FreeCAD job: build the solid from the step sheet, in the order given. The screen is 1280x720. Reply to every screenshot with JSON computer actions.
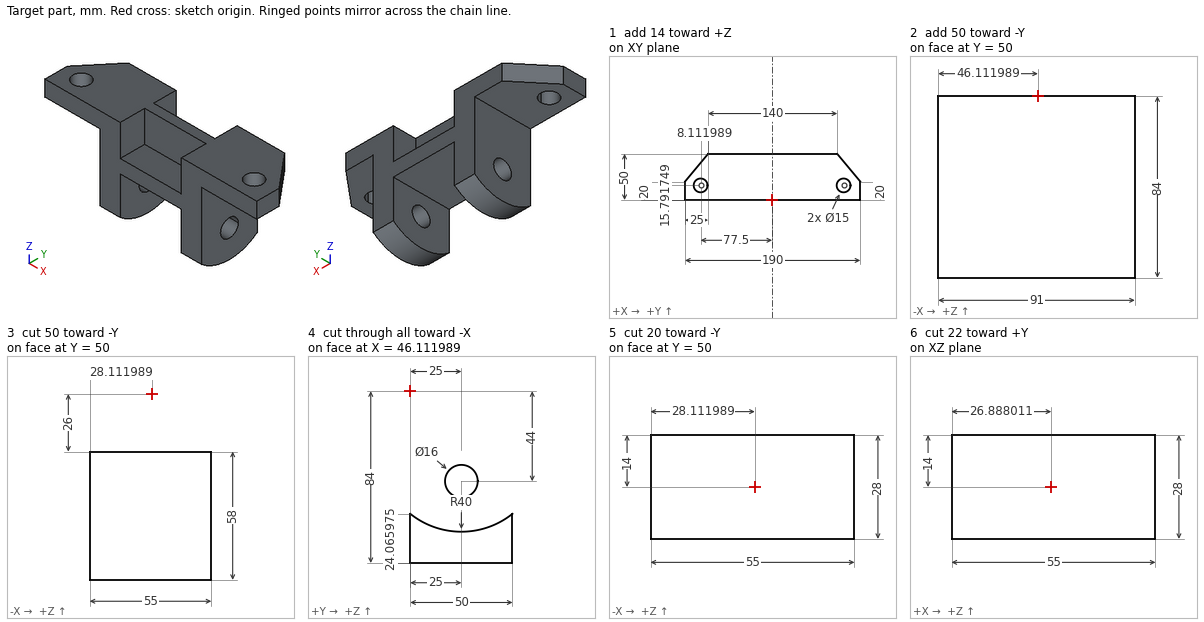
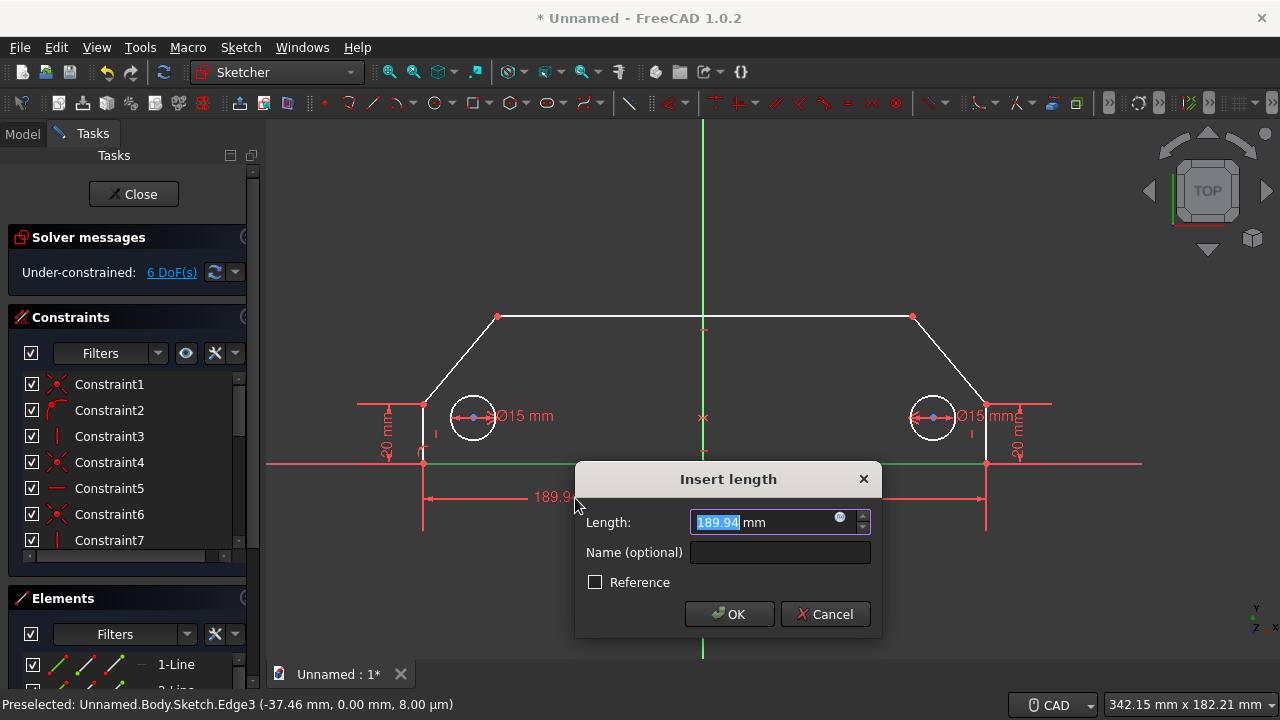
{"action": "type", "text": "190"}
{"action": "key", "text": "Return"}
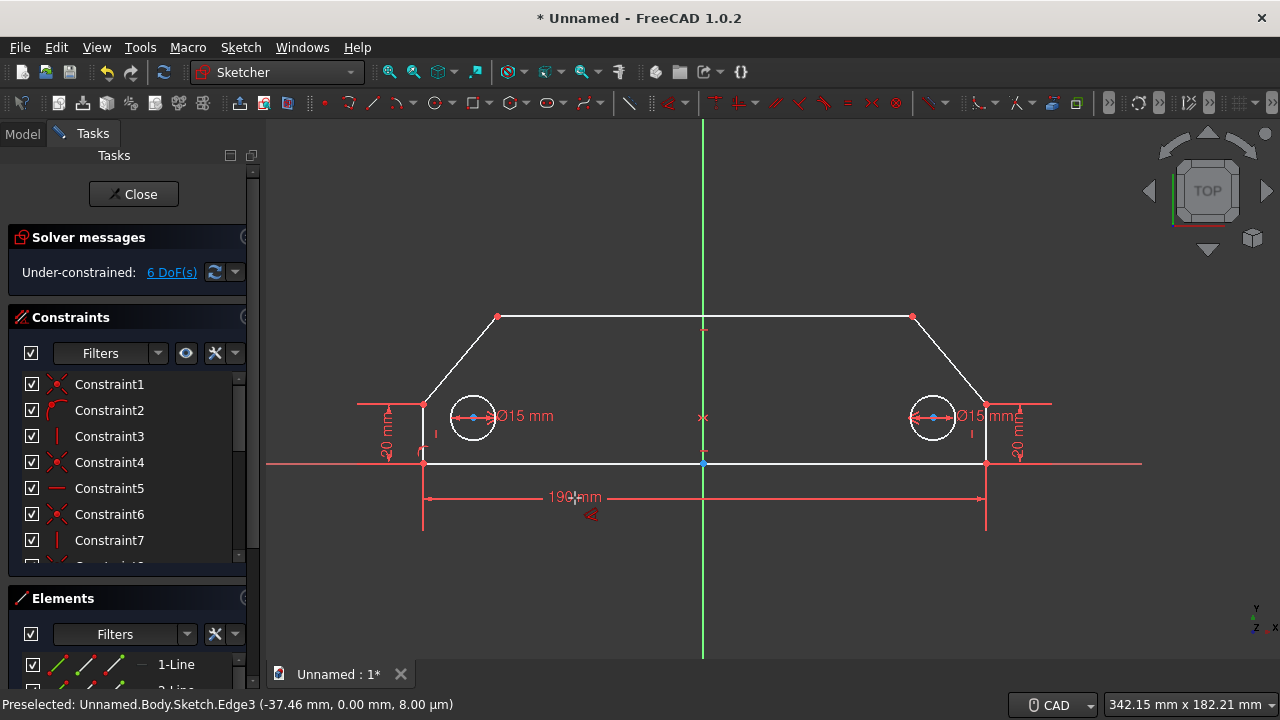
{"action": "left_click", "coordinate": [788, 316]}
{"action": "left_click", "coordinate": [609, 282]}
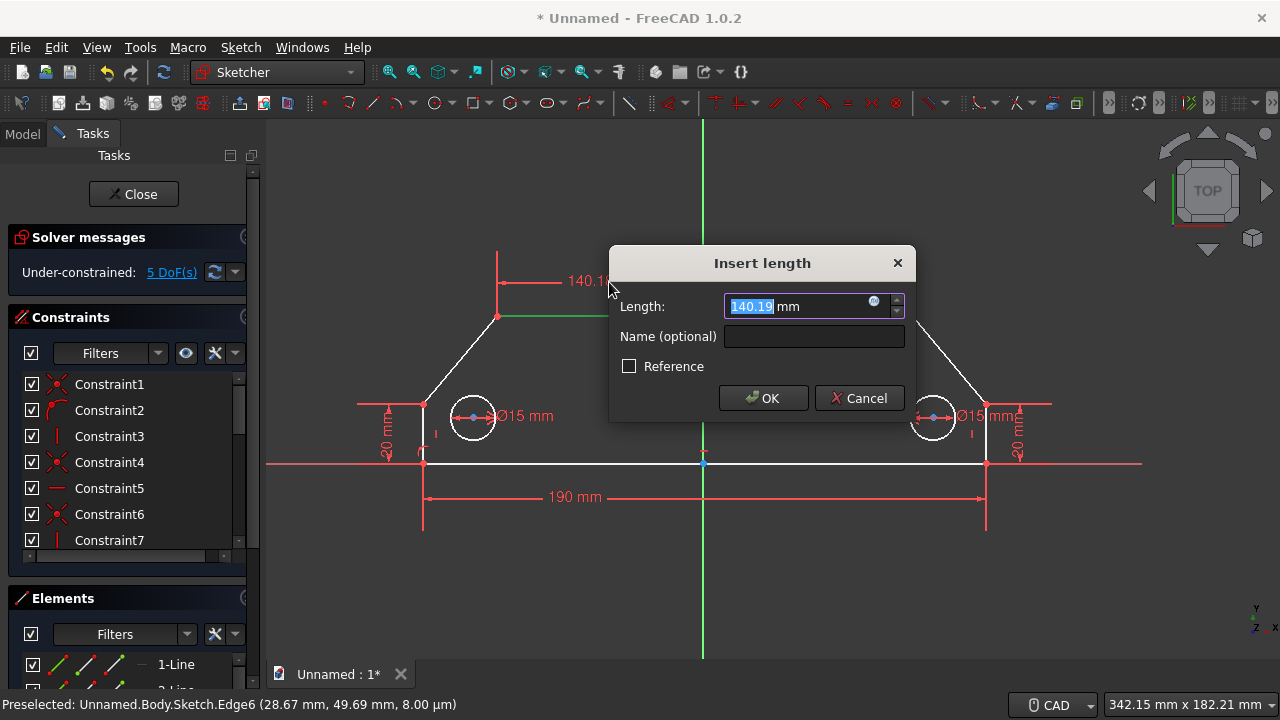
{"action": "type", "text": "140"}
{"action": "key", "text": "Return"}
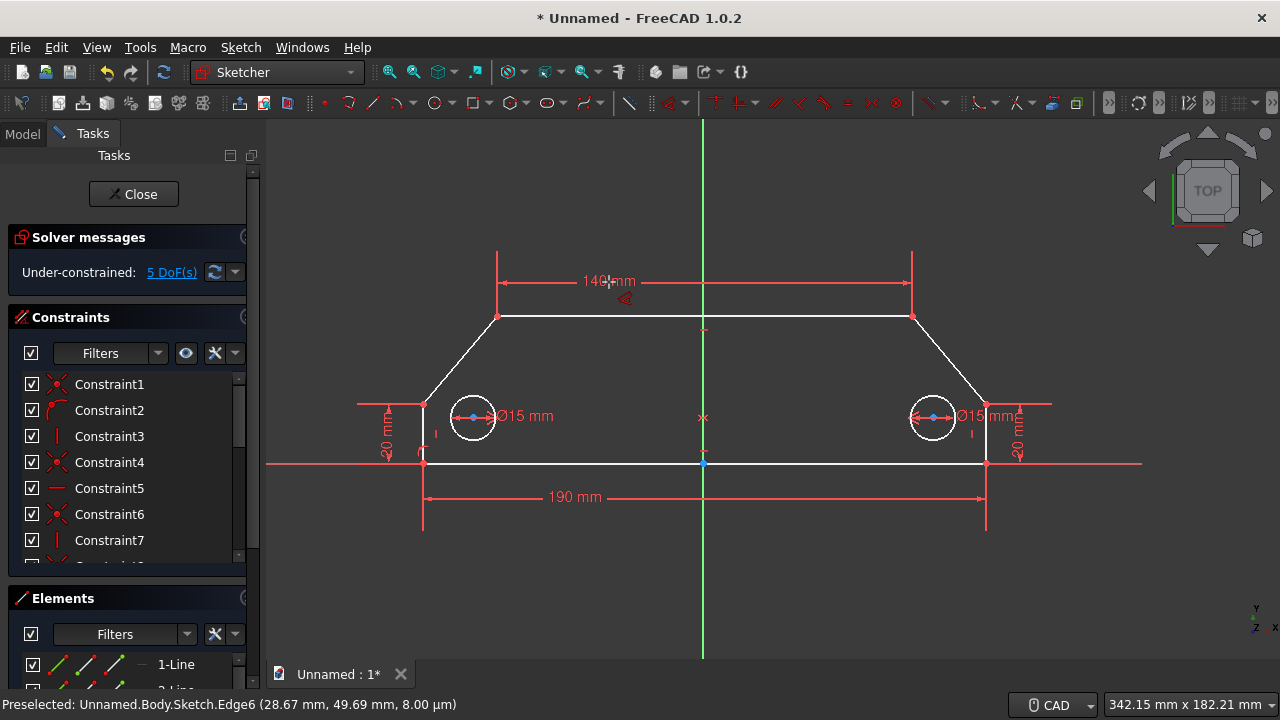
{"action": "left_click", "coordinate": [497, 316]}
{"action": "left_click", "coordinate": [737, 390]}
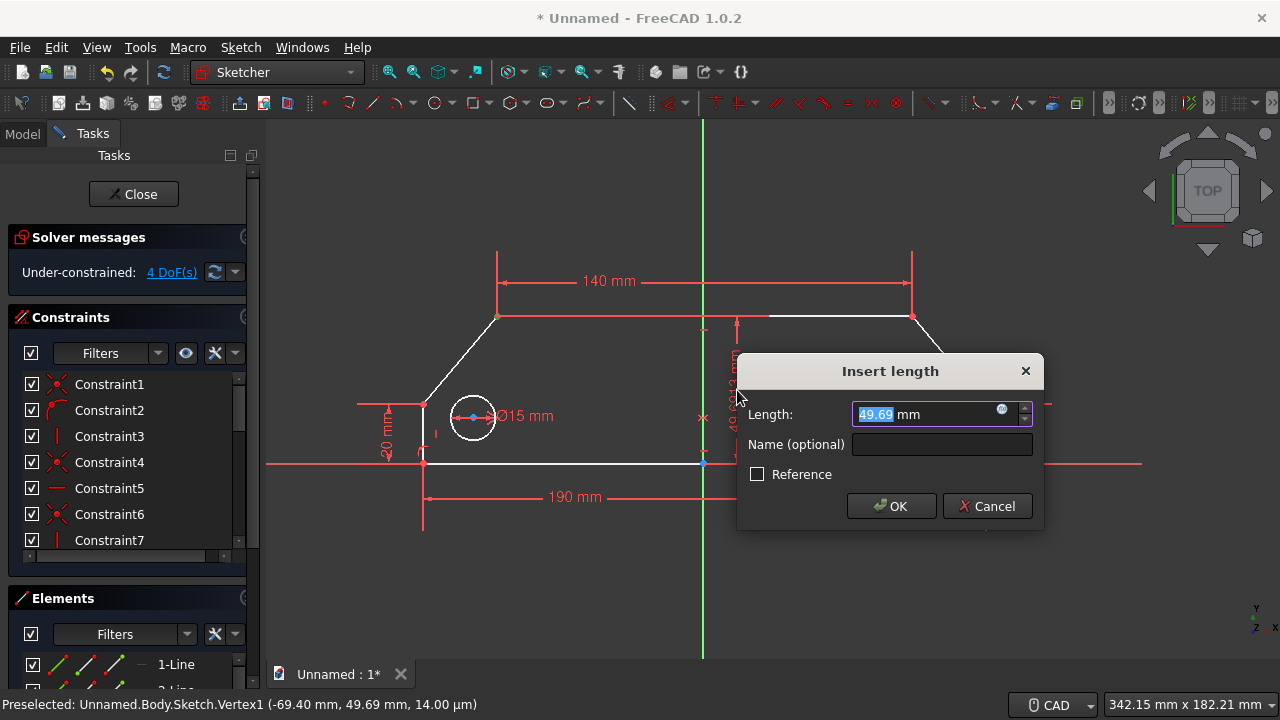
{"action": "type", "text": "50"}
{"action": "key", "text": "Return"}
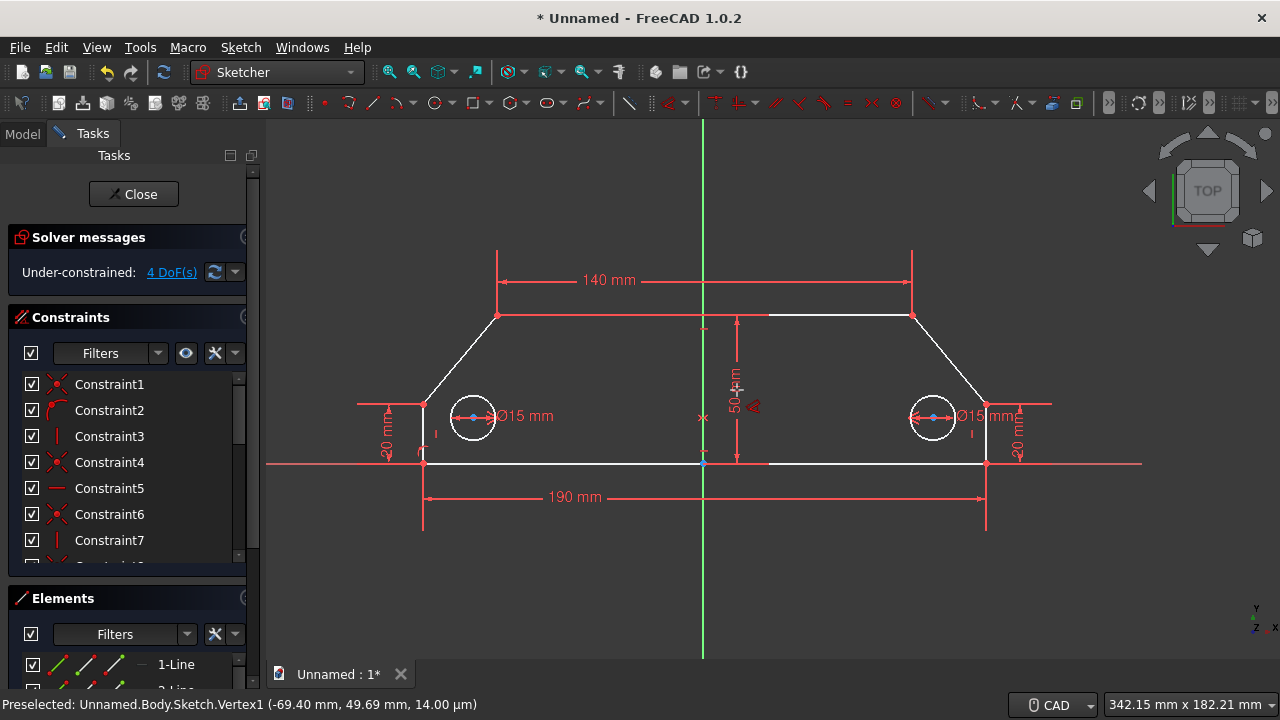
{"action": "left_click", "coordinate": [475, 342]}
{"action": "left_click", "coordinate": [460, 281]}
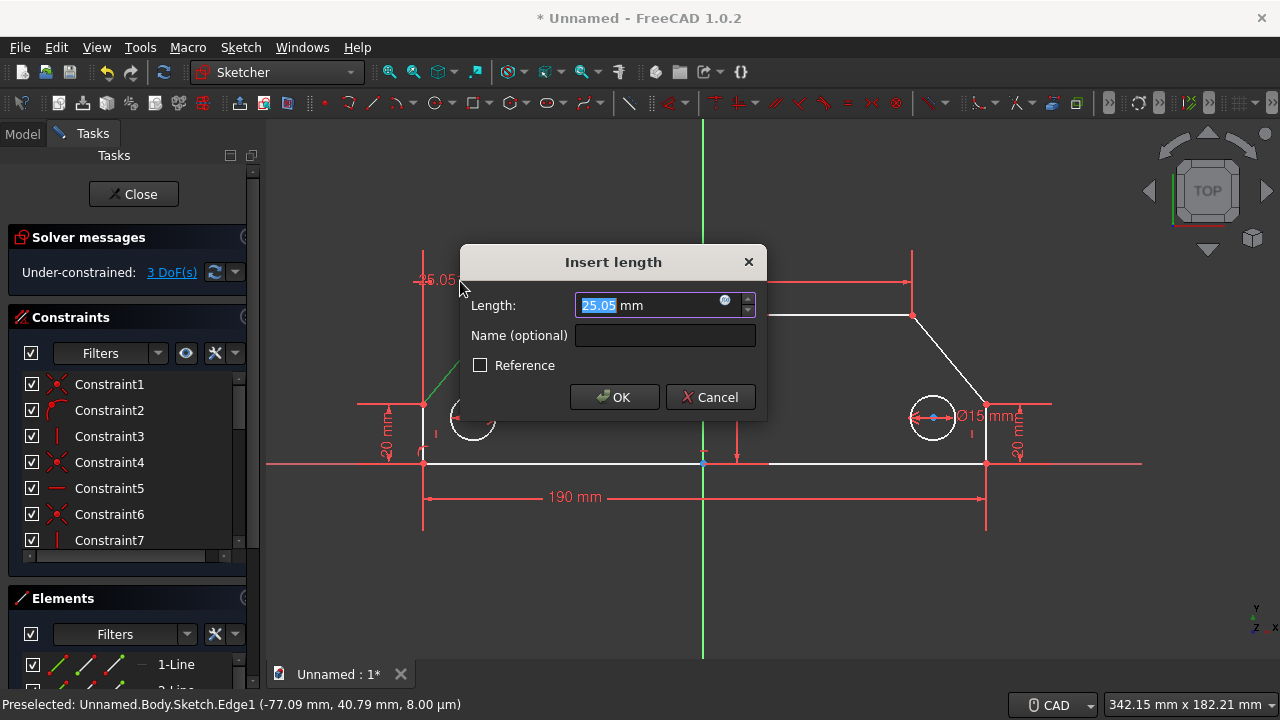
{"action": "type", "text": "25"}
{"action": "key", "text": "Return"}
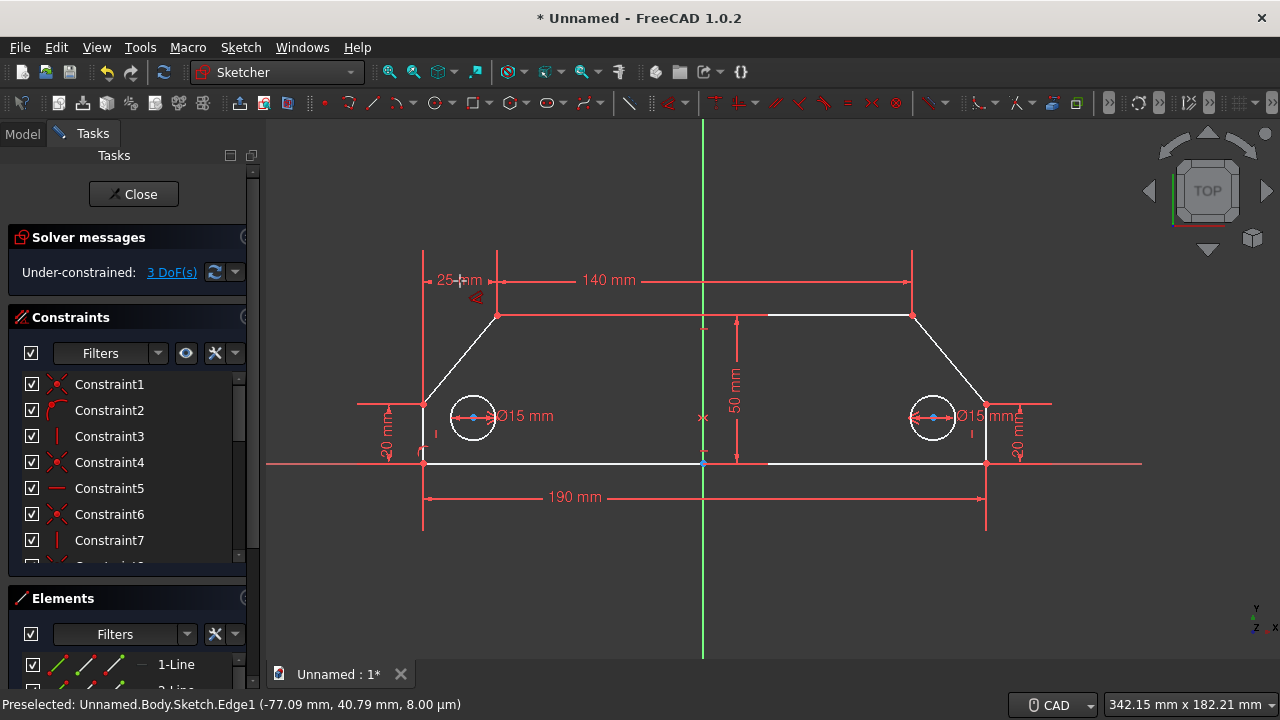
{"action": "left_click", "coordinate": [473, 418]}
{"action": "left_click", "coordinate": [669, 498]}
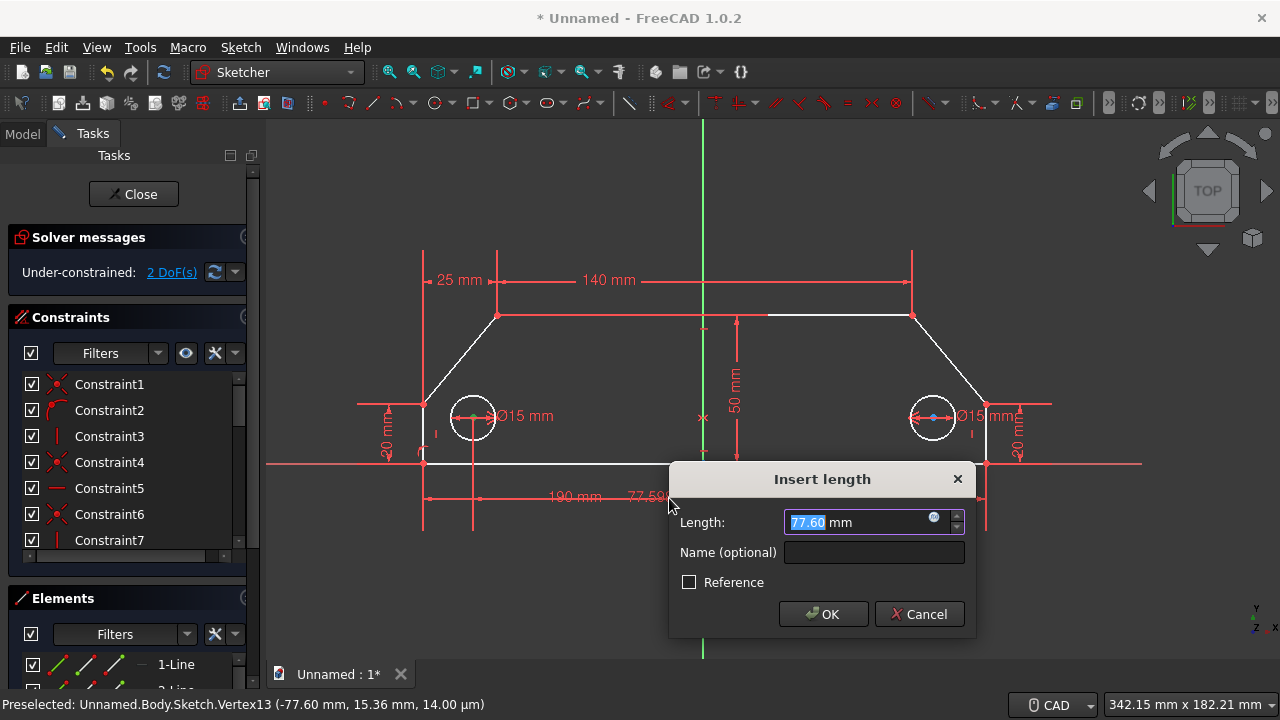
{"action": "type", "text": "77.5"}
{"action": "key", "text": "Return"}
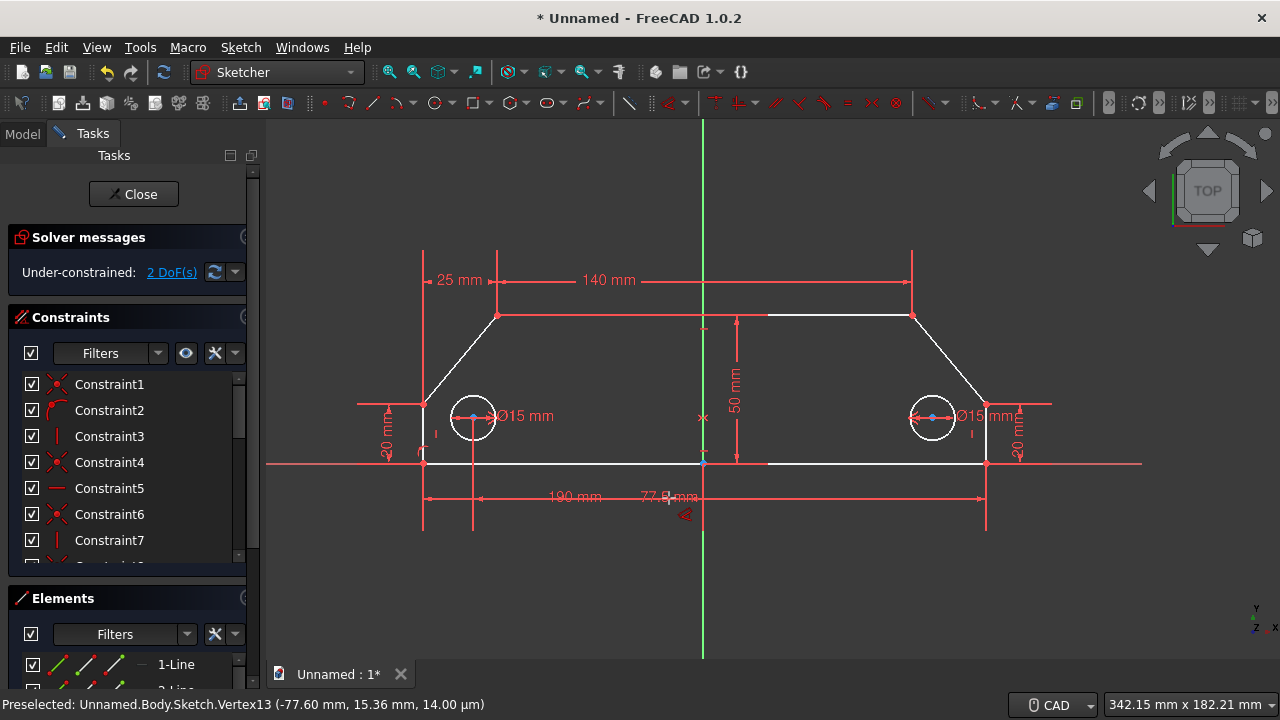
{"action": "left_click", "coordinate": [473, 418]}
{"action": "left_click", "coordinate": [737, 441]}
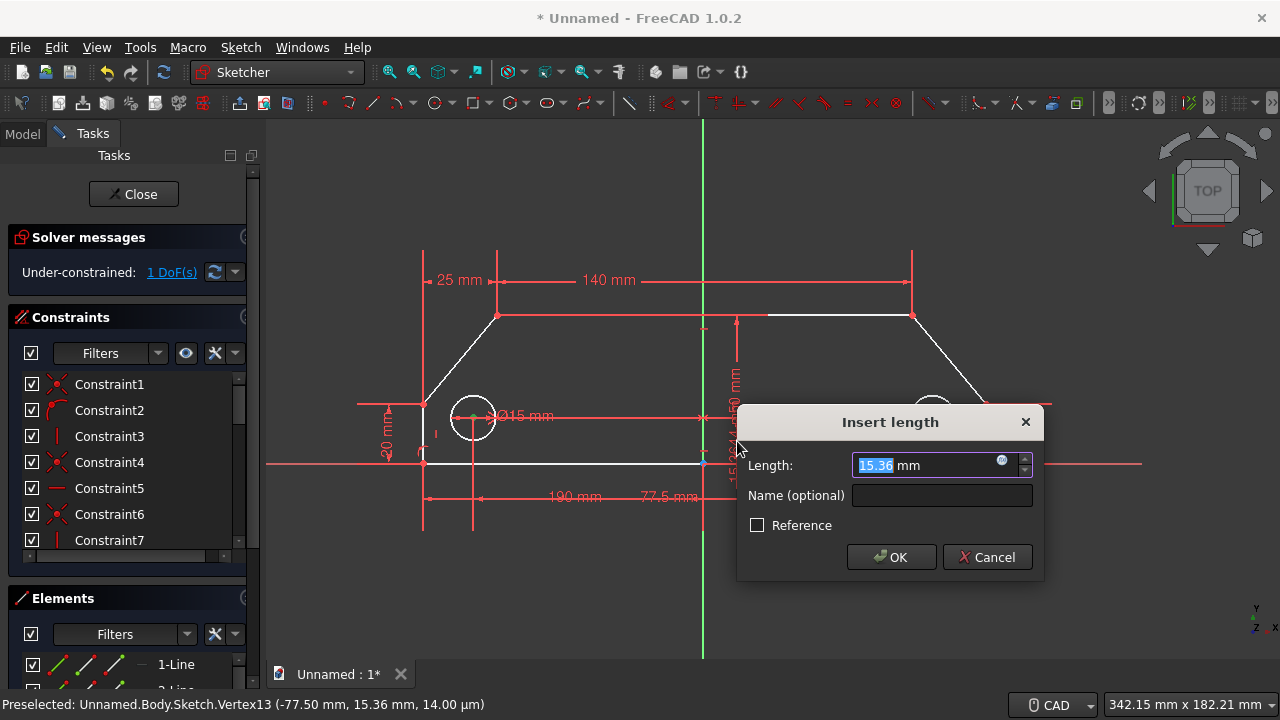
{"action": "type", "text": "15.791749"}
{"action": "key", "text": "Return"}